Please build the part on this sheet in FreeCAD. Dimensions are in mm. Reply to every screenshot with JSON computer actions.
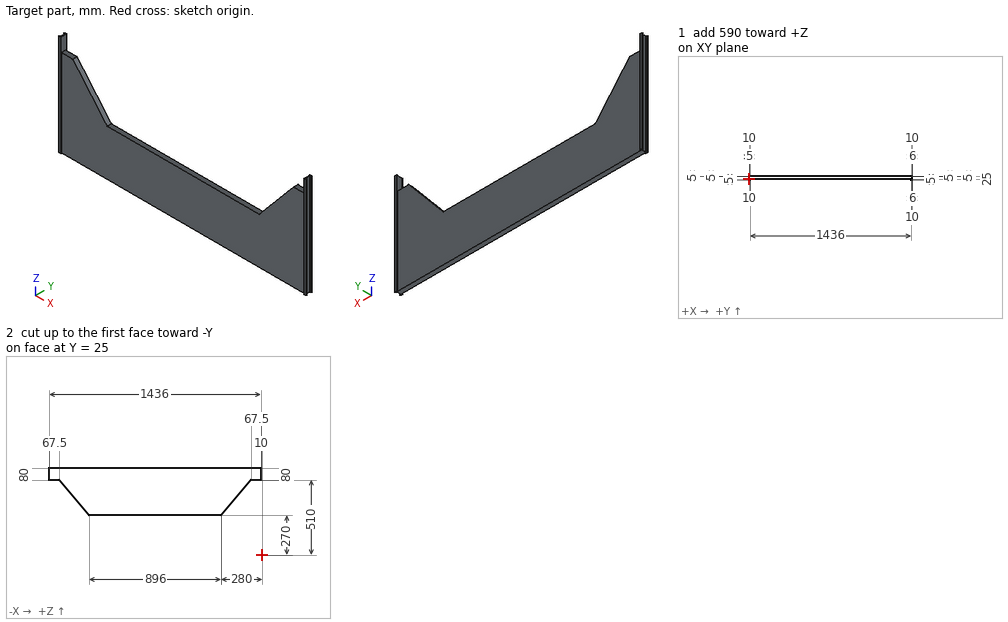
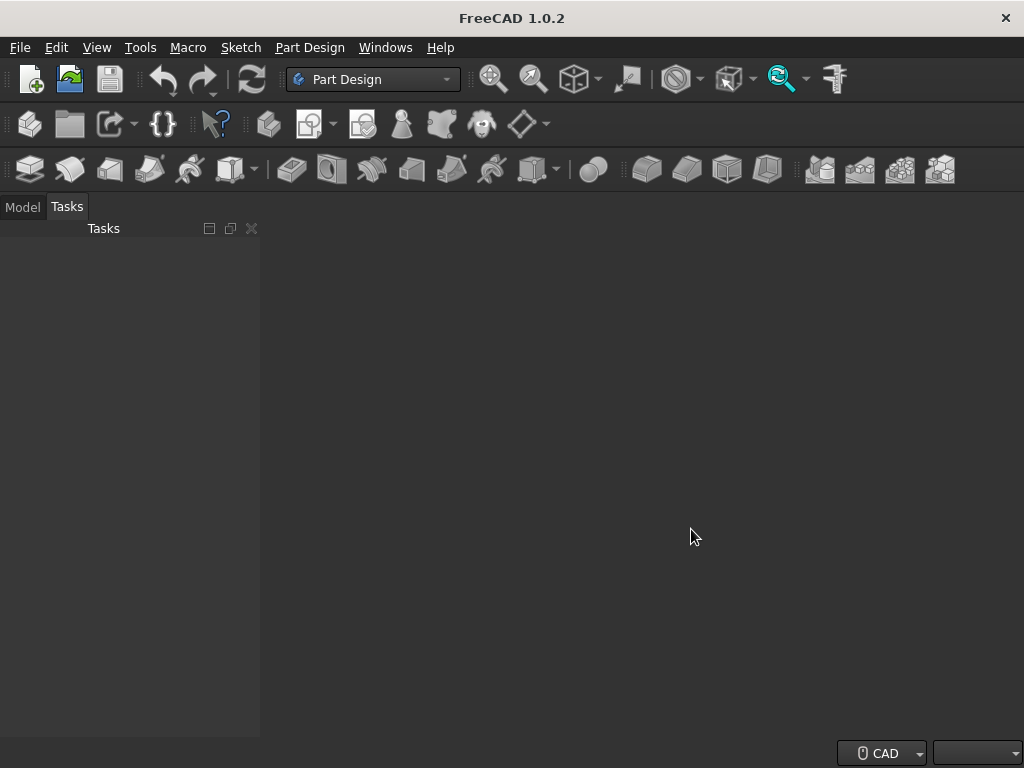
{"action": "key", "text": "ctrl+n"}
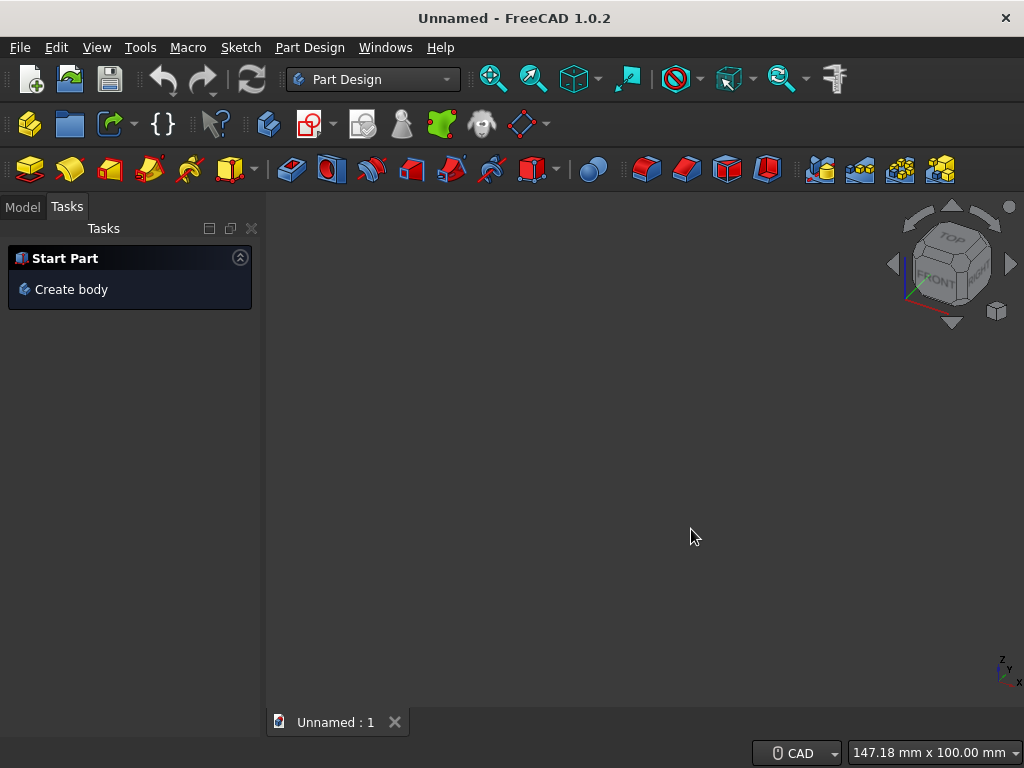
{"action": "left_click", "coordinate": [310, 124]}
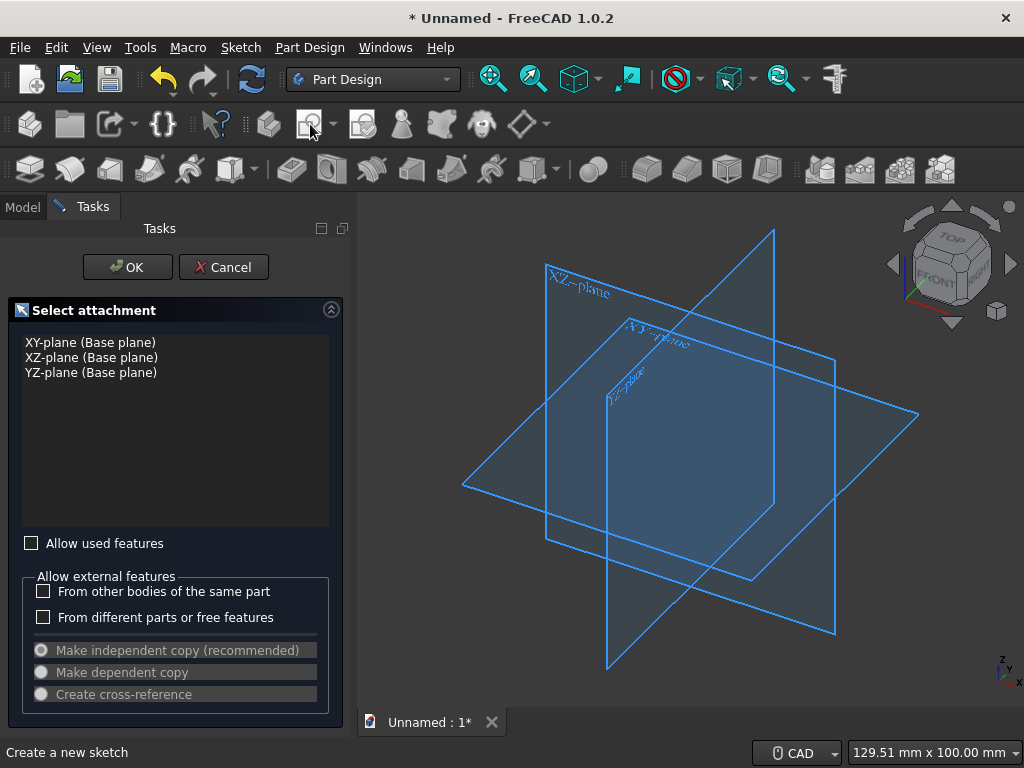
{"action": "left_click", "coordinate": [82, 342]}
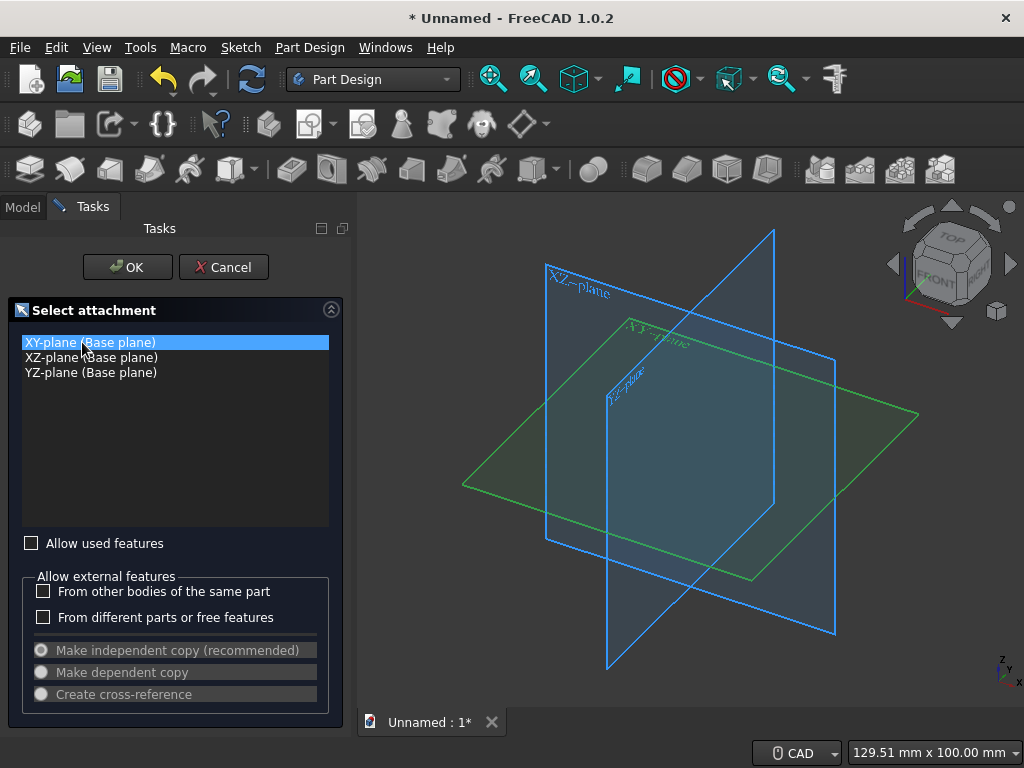
{"action": "left_click", "coordinate": [128, 267]}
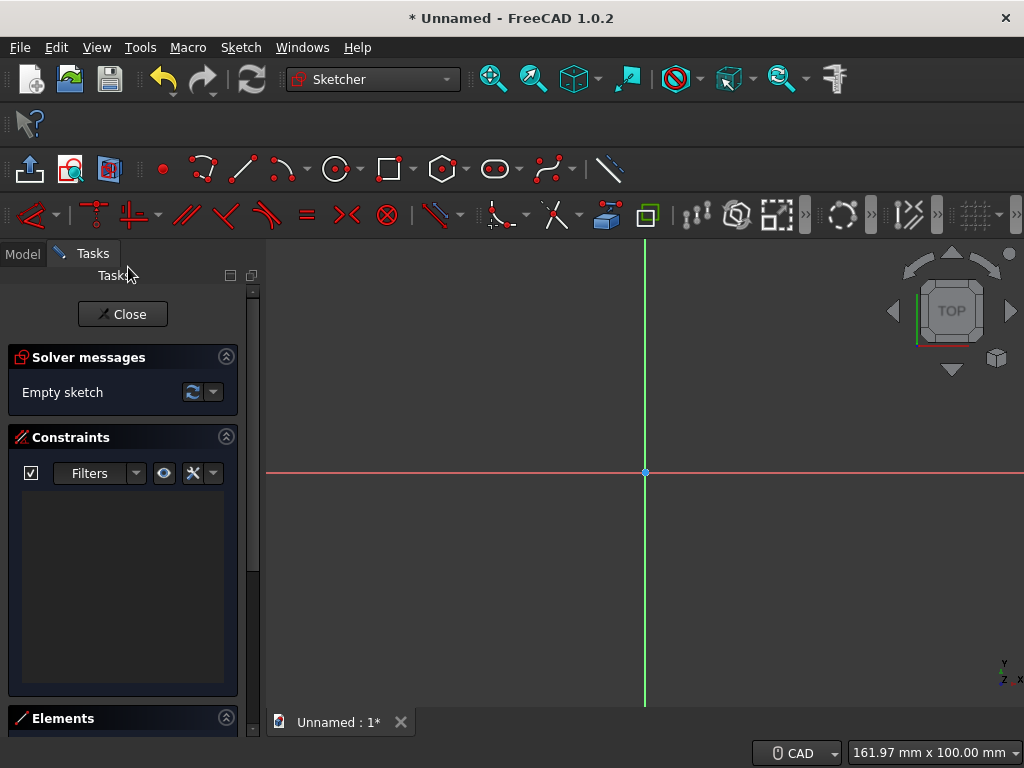
{"action": "scroll", "coordinate": [351, 477], "scroll_direction": "down", "scroll_amount": 14}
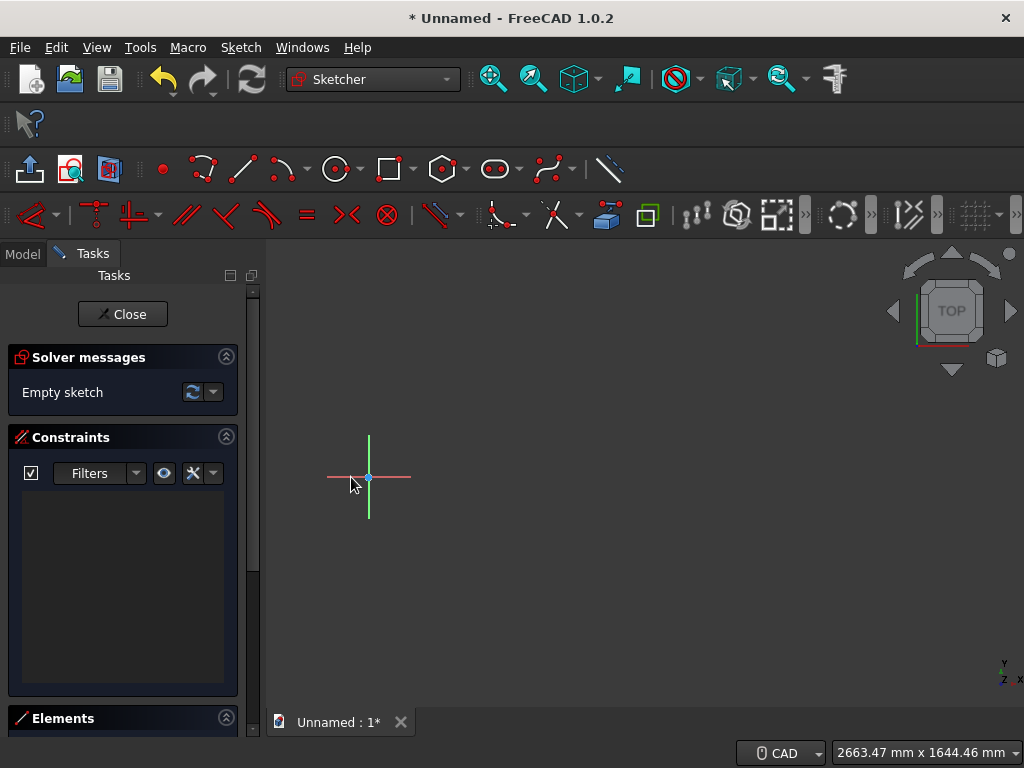
{"action": "key", "text": "g m"}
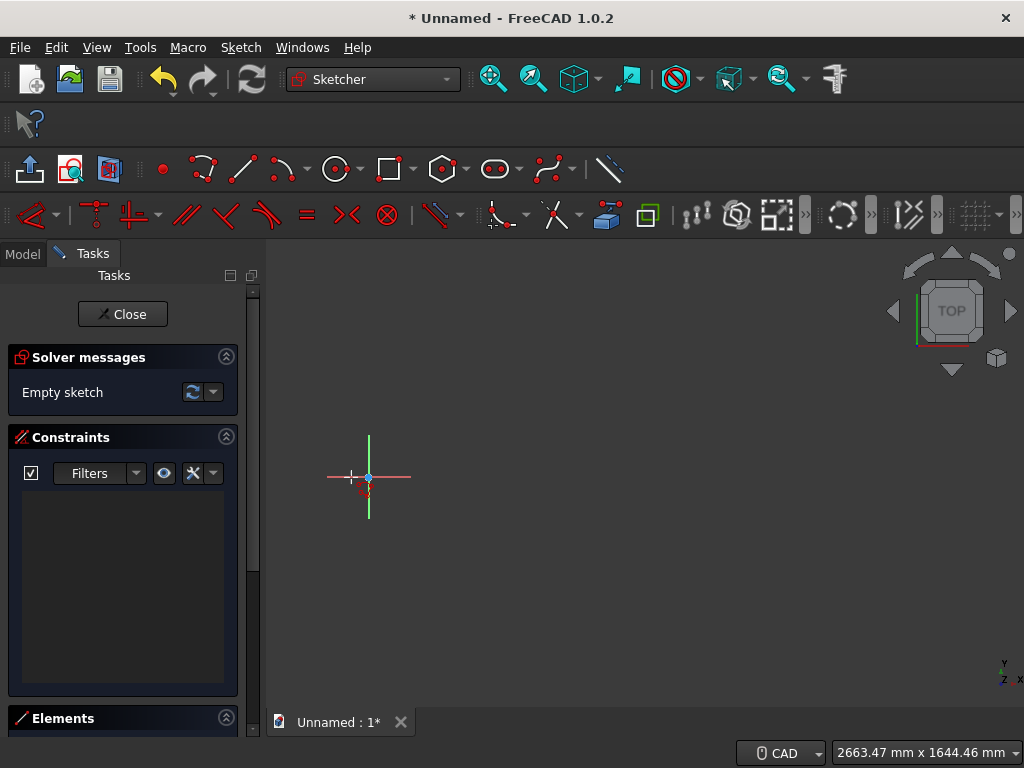
{"action": "left_click", "coordinate": [369, 477]}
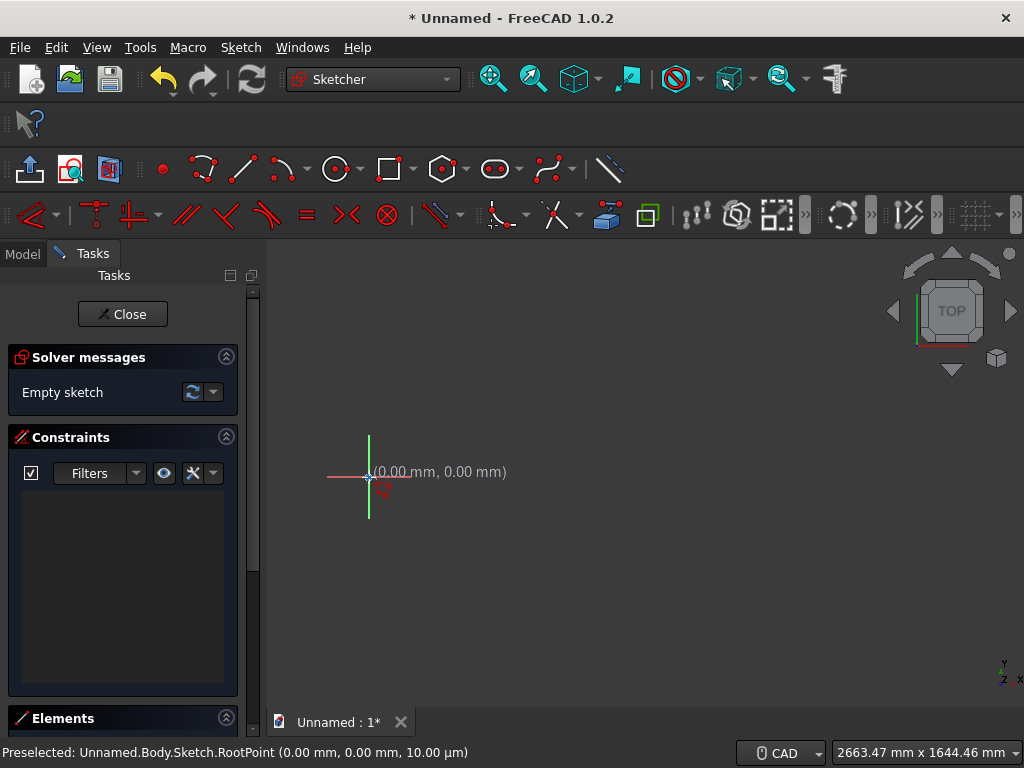
{"action": "scroll", "coordinate": [369, 479], "scroll_direction": "up", "scroll_amount": 13}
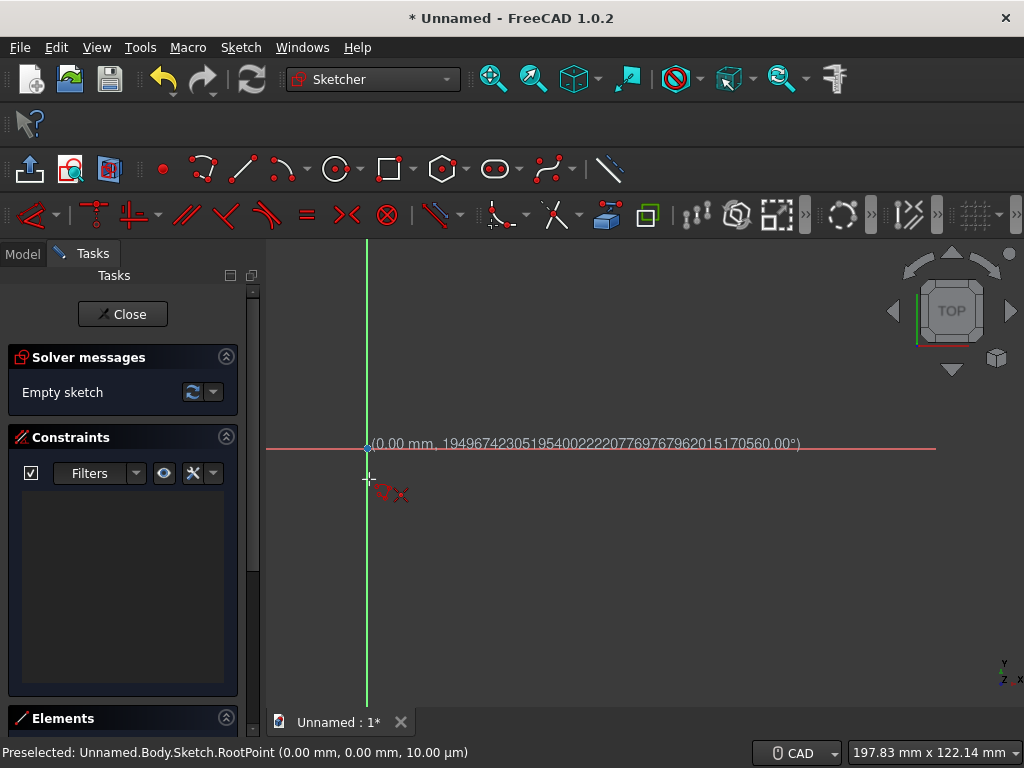
{"action": "left_click", "coordinate": [376, 468]}
{"action": "left_click", "coordinate": [405, 468]}
{"action": "left_click", "coordinate": [405, 449]}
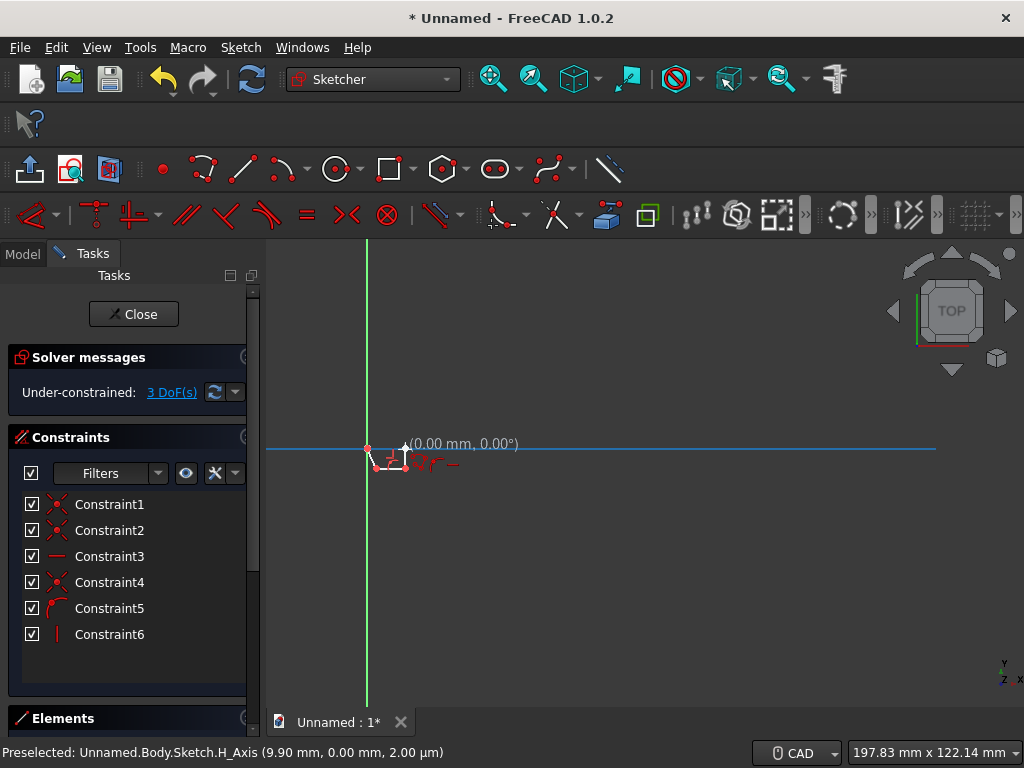
{"action": "scroll", "coordinate": [369, 479], "scroll_direction": "down", "scroll_amount": 13}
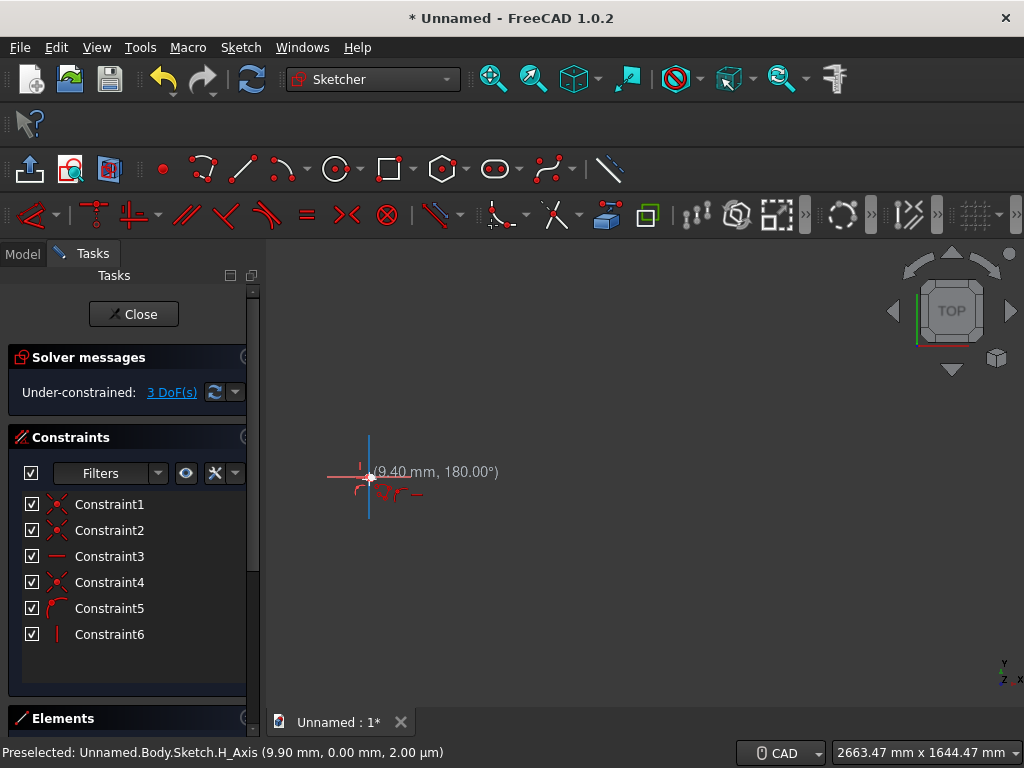
{"action": "left_click", "coordinate": [781, 468]}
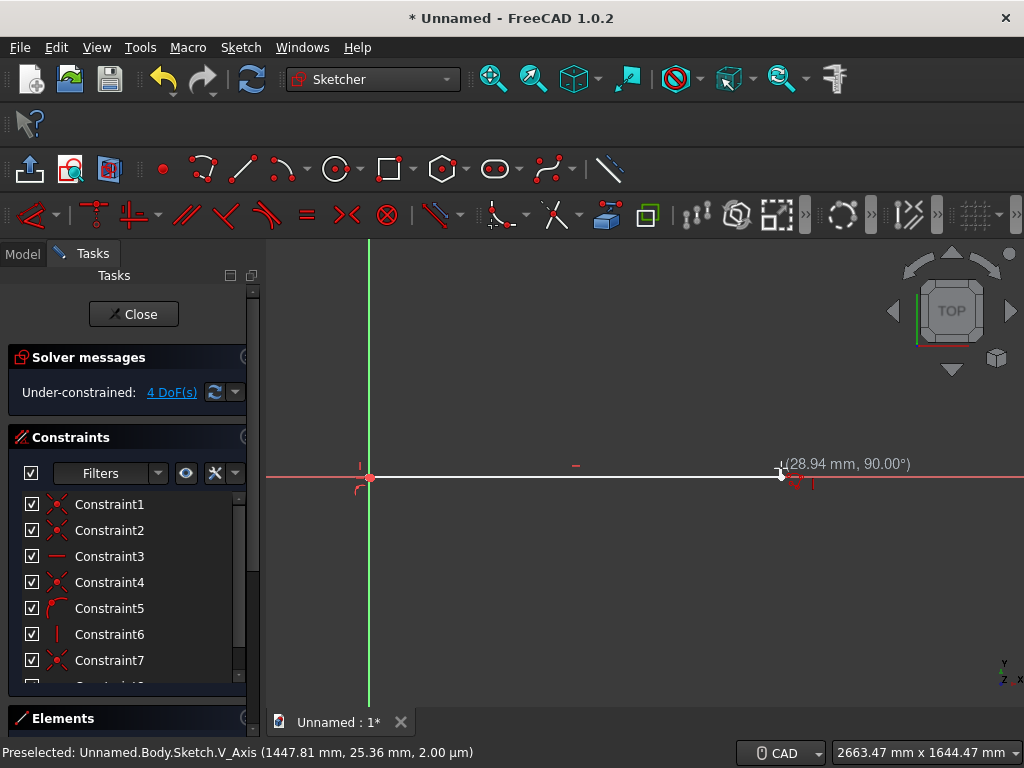
{"action": "scroll", "coordinate": [781, 479], "scroll_direction": "up", "scroll_amount": 13}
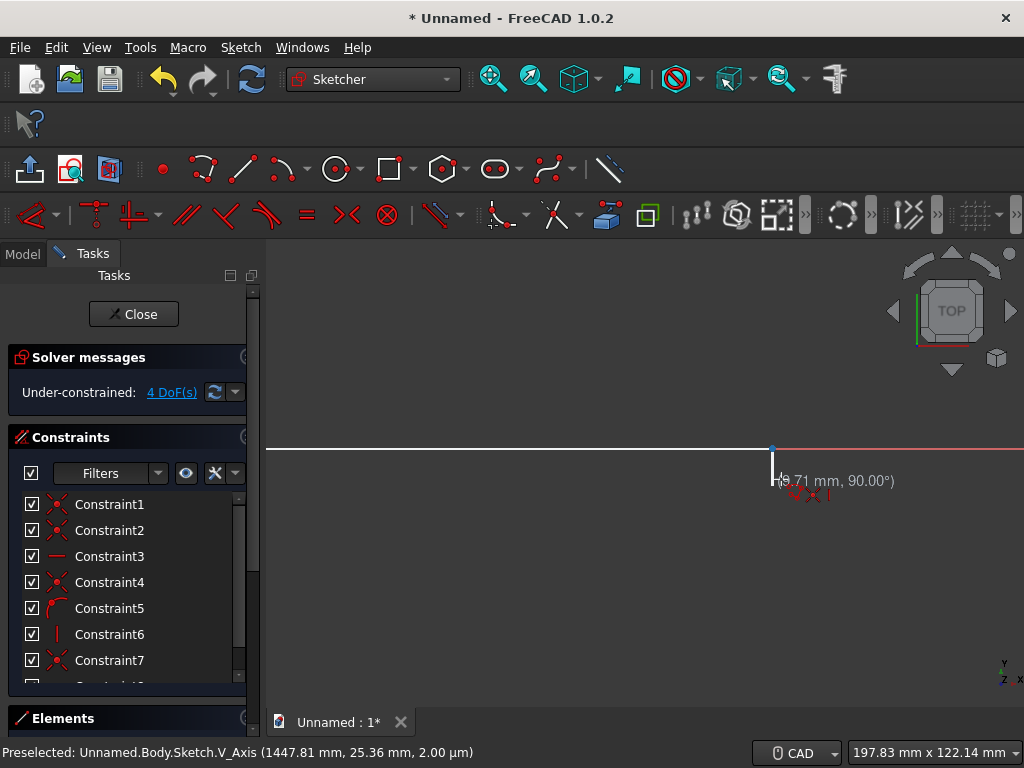
{"action": "left_click", "coordinate": [773, 468]}
{"action": "left_click", "coordinate": [804, 468]}
{"action": "left_click", "coordinate": [804, 449]}
{"action": "left_click", "coordinate": [781, 440]}